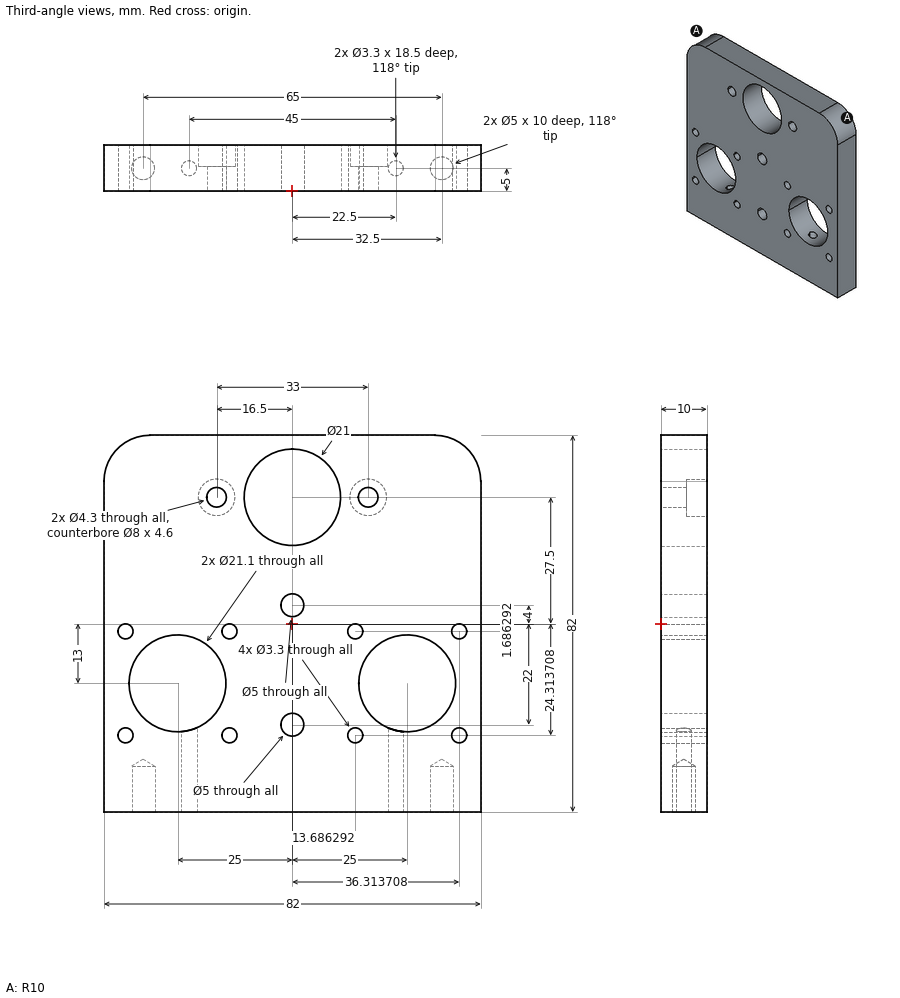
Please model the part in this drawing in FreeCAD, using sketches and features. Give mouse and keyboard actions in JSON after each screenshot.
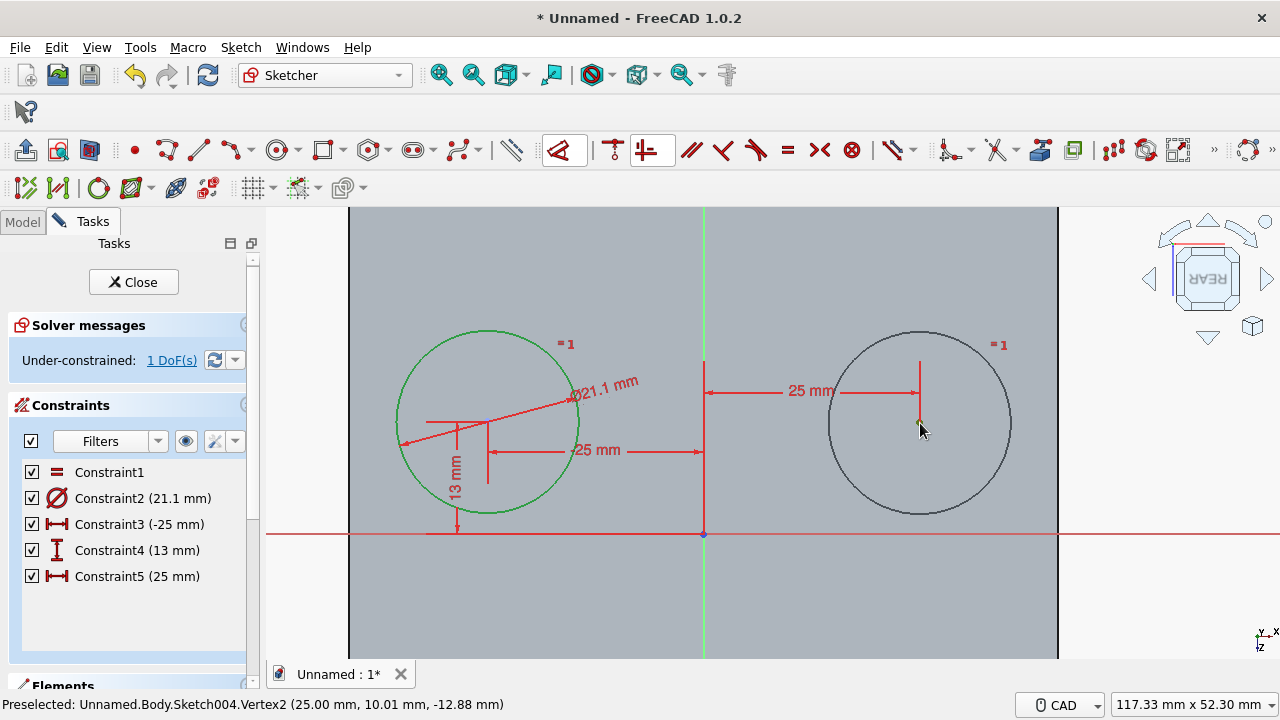
{"action": "key", "text": "i"}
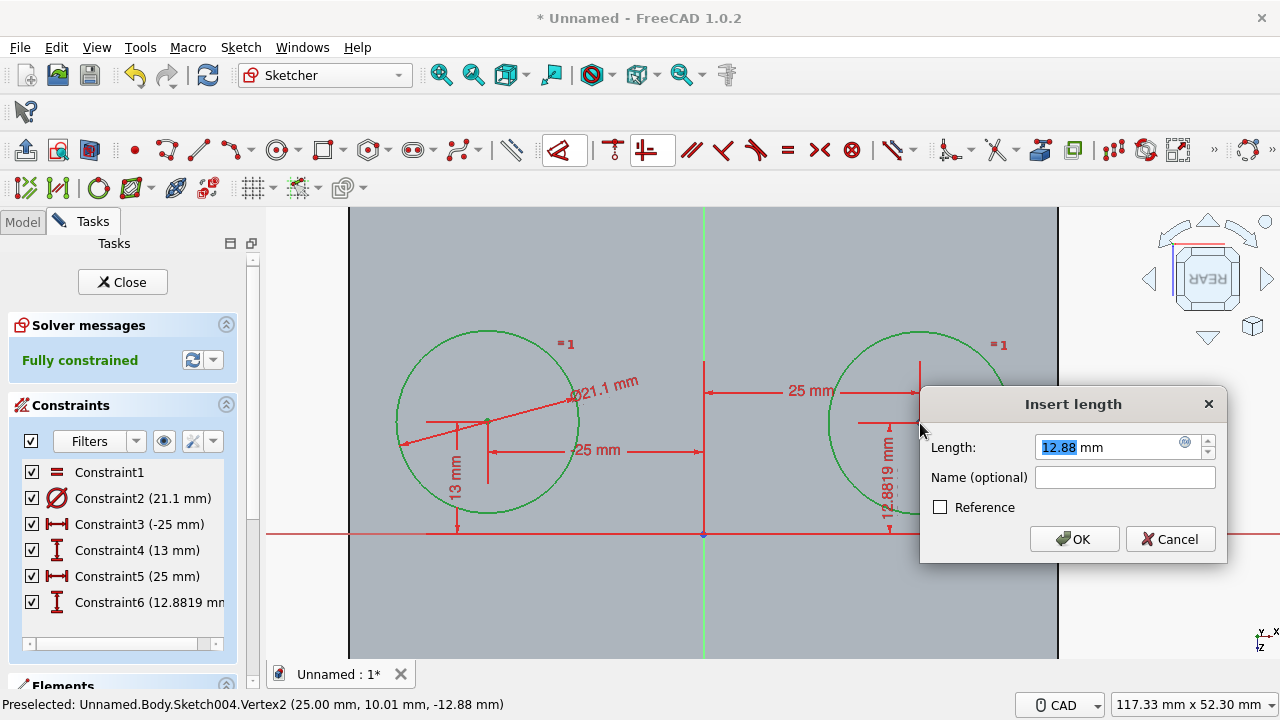
{"action": "type", "text": "13"}
{"action": "key", "text": "Return"}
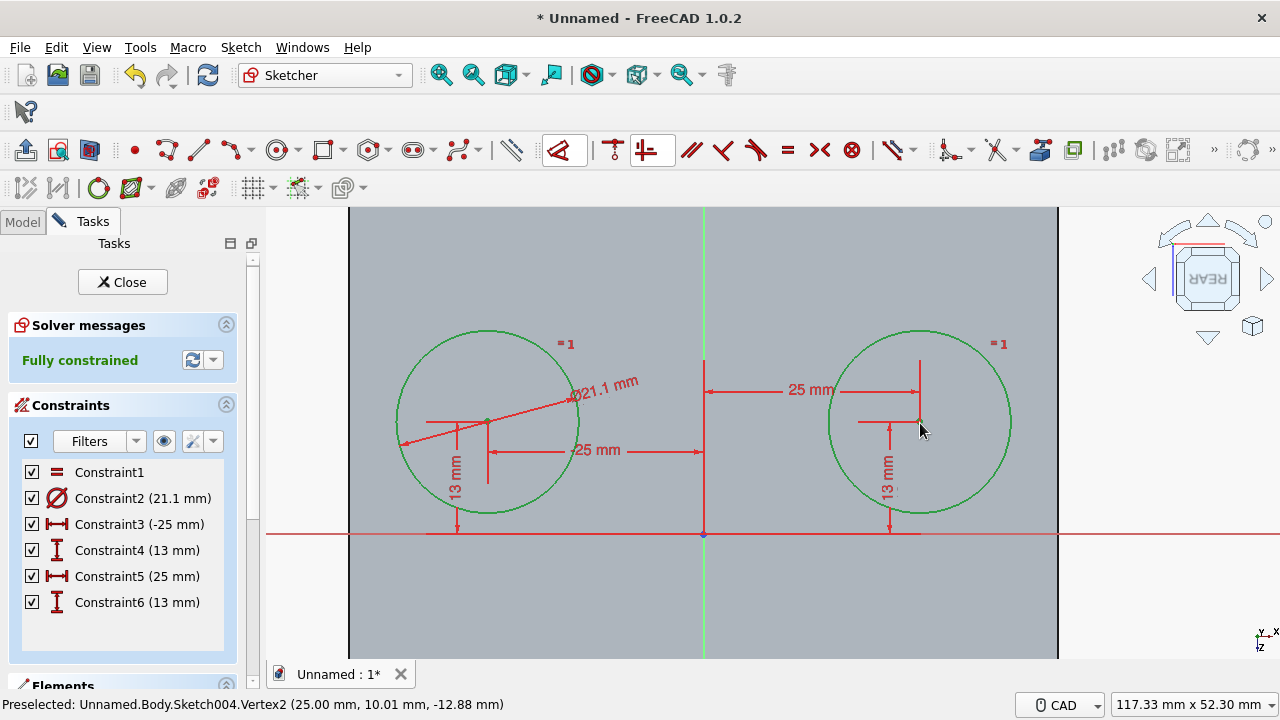
{"action": "left_click", "coordinate": [123, 282]}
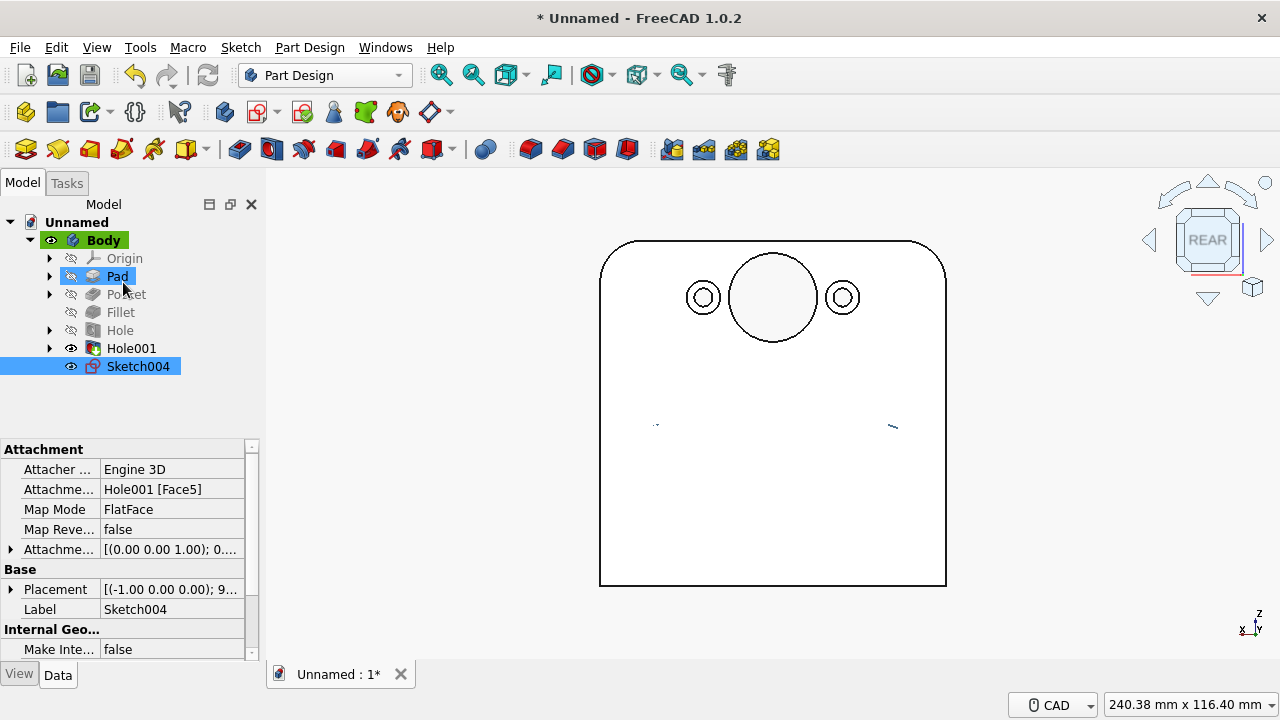
{"action": "left_click", "coordinate": [272, 150]}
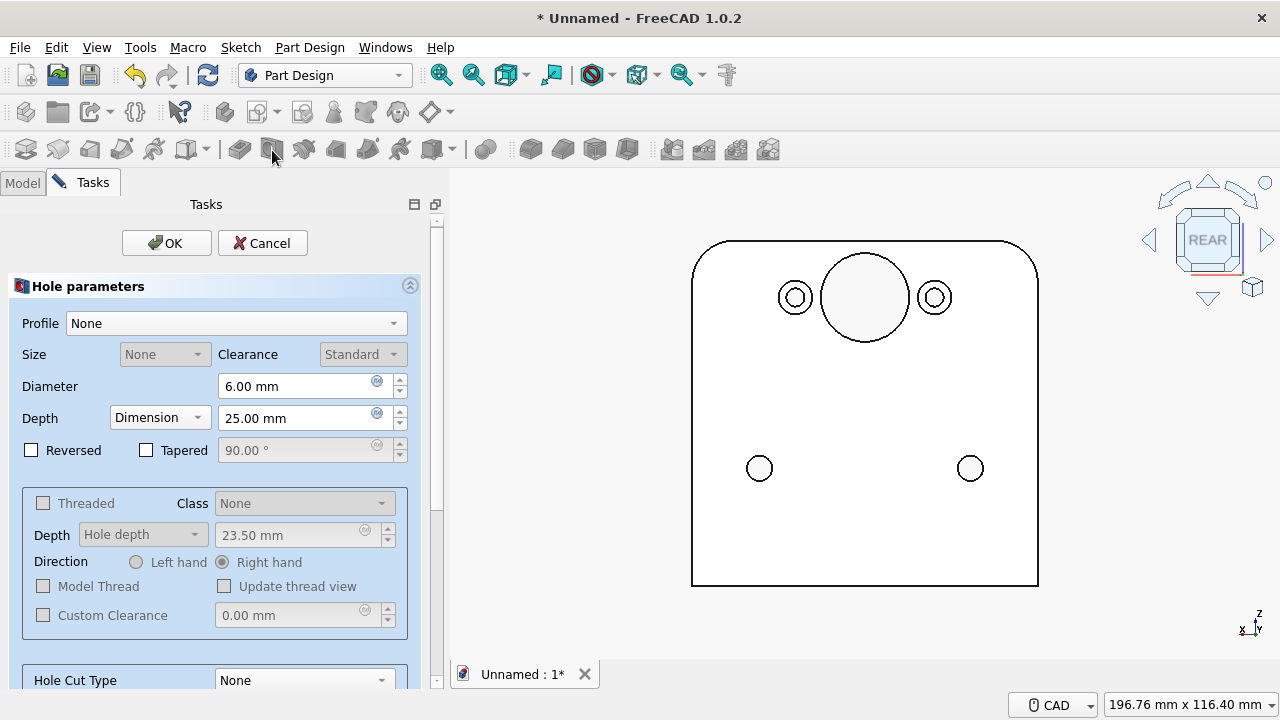
{"action": "triple_click", "coordinate": [305, 386]}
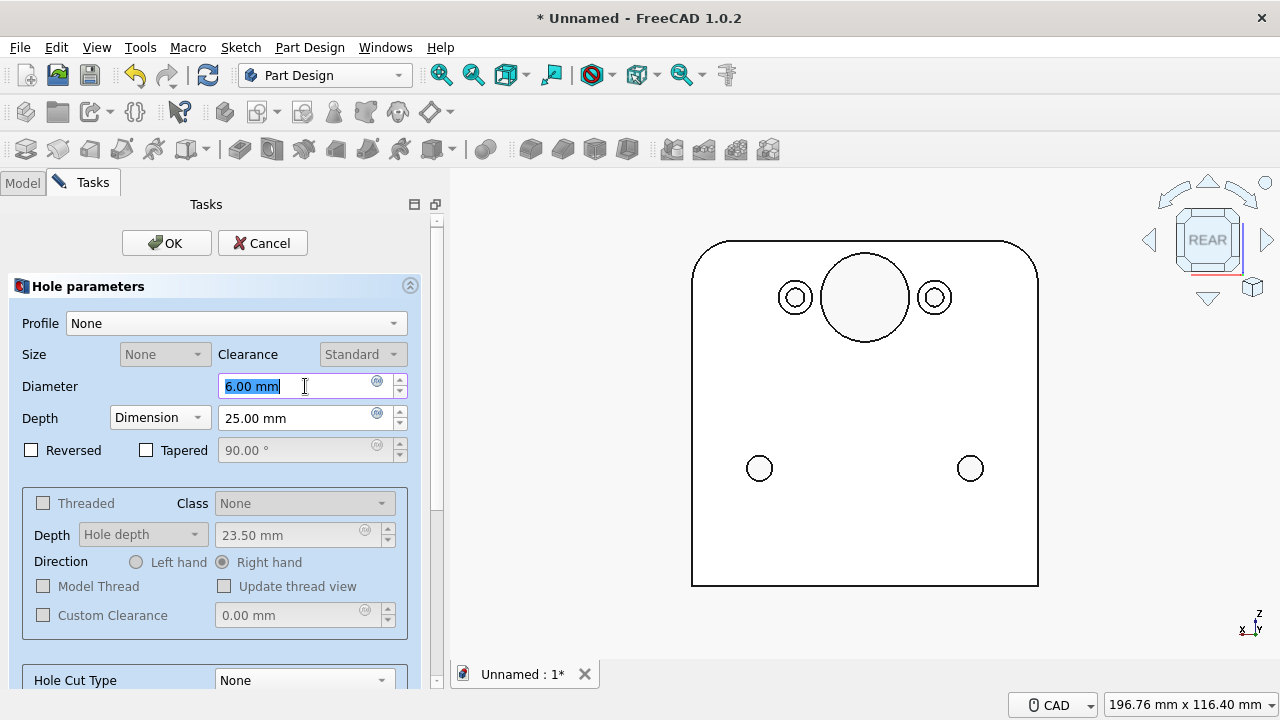
{"action": "type", "text": "21.1"}
{"action": "key", "text": "Tab"}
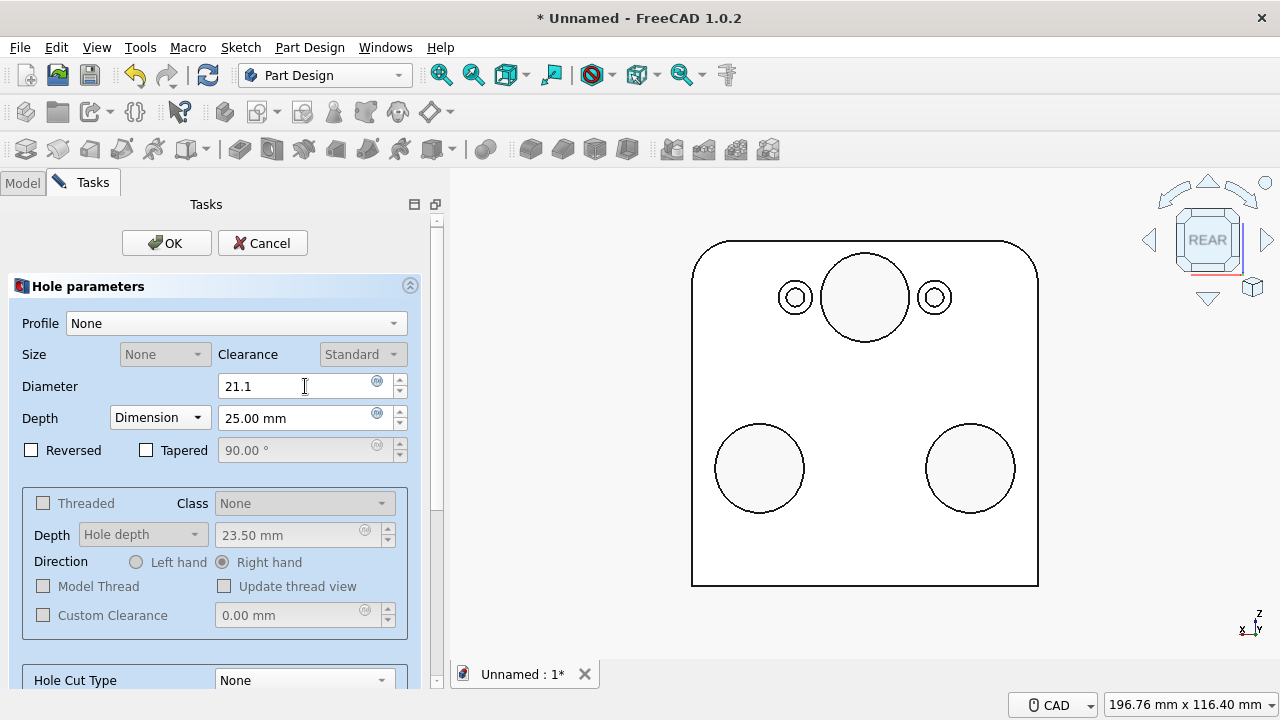
{"action": "left_click", "coordinate": [161, 418]}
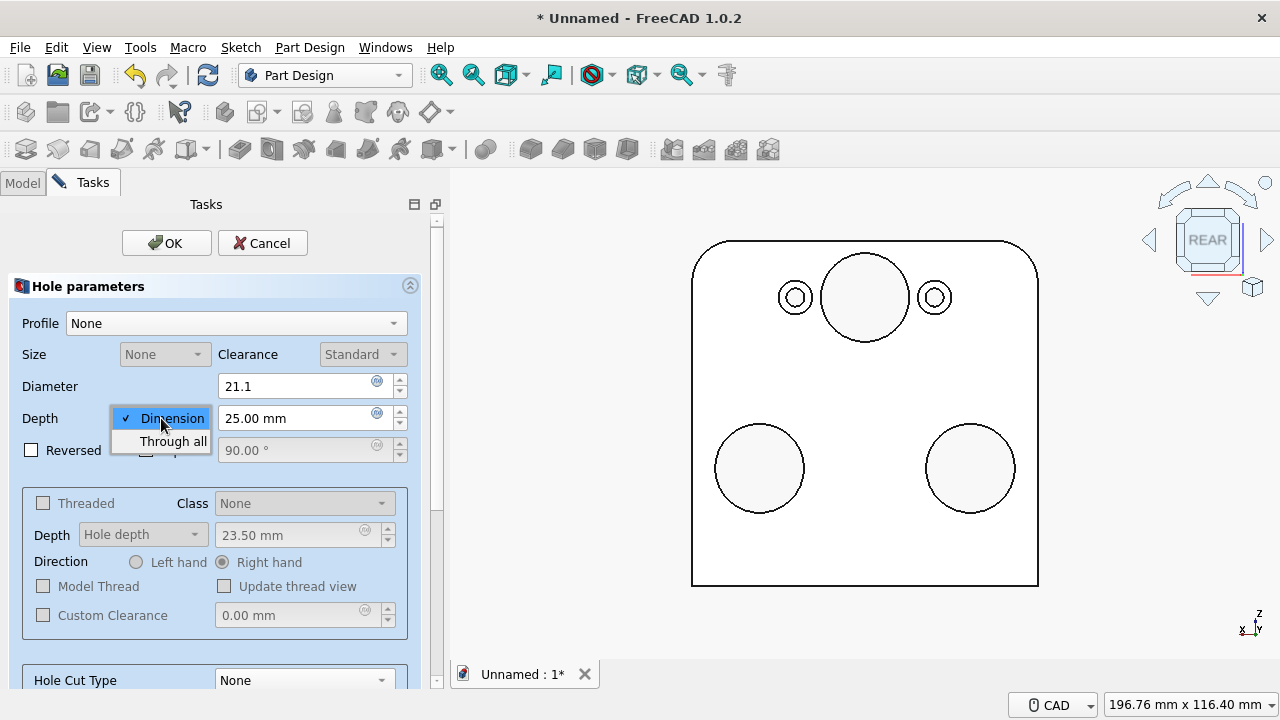
{"action": "left_click", "coordinate": [160, 442]}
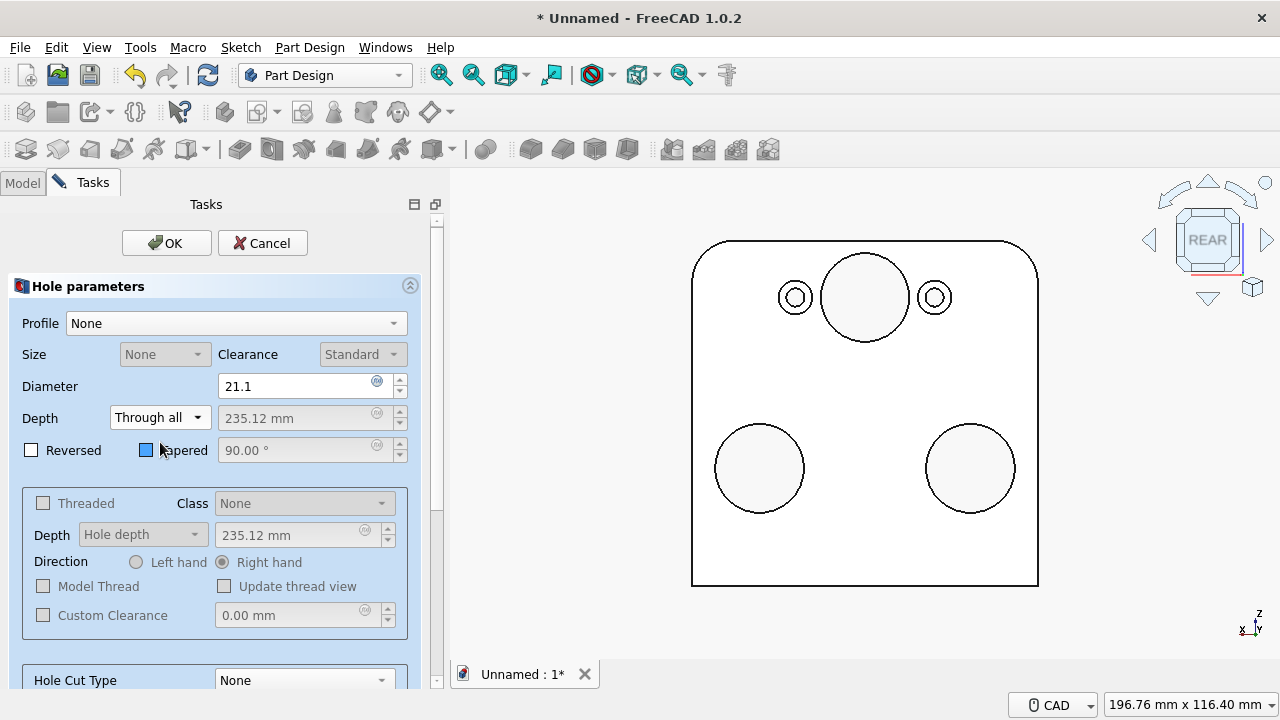
{"action": "left_click", "coordinate": [167, 243]}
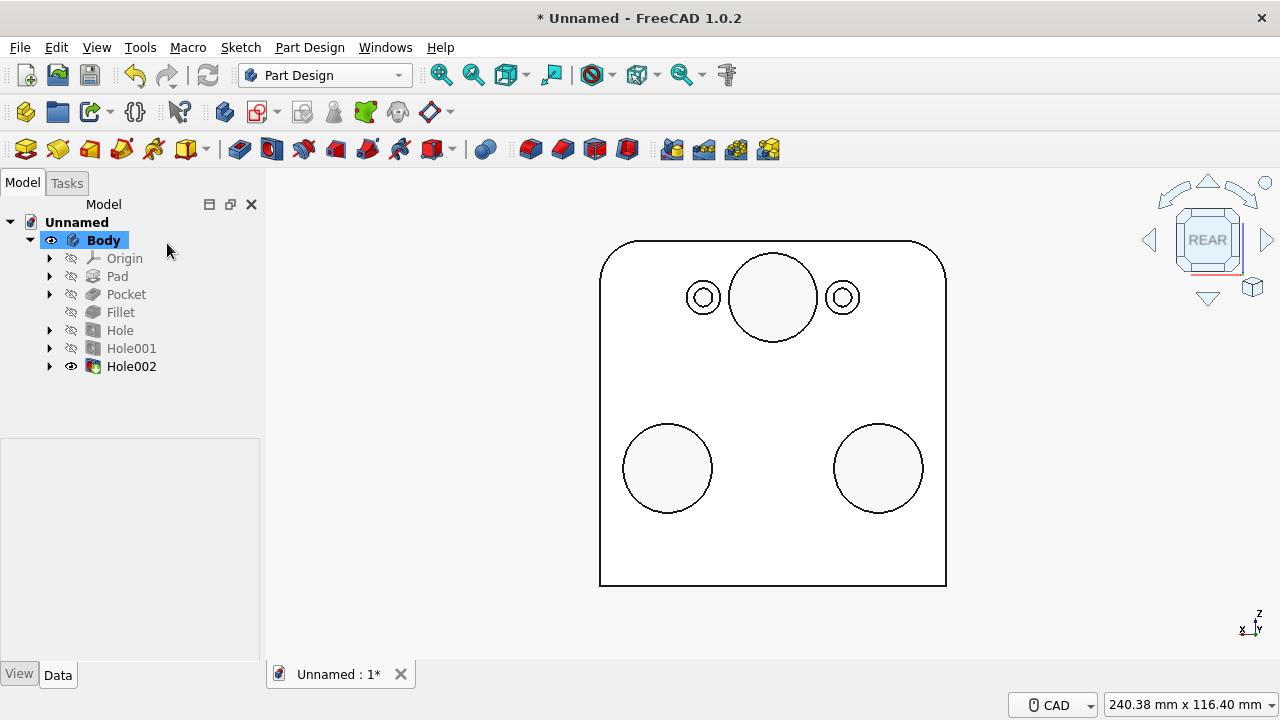
{"action": "left_click", "coordinate": [258, 112]}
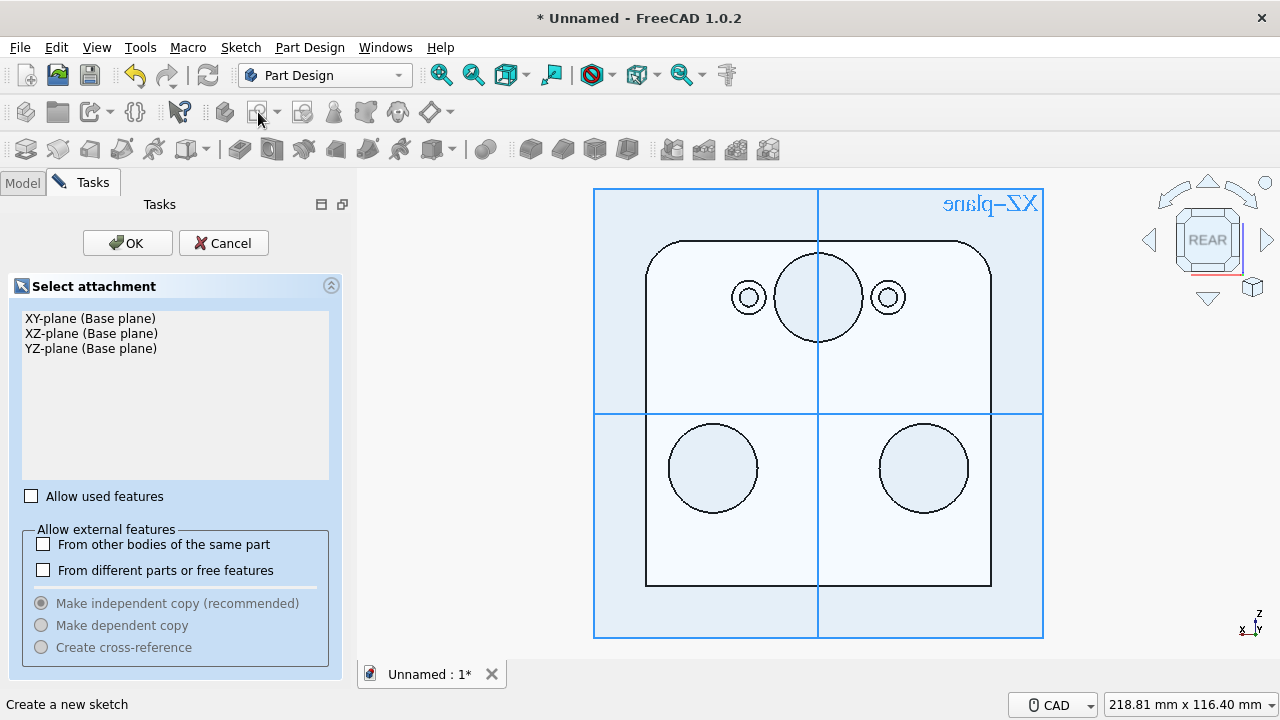
{"action": "left_click", "coordinate": [82, 334]}